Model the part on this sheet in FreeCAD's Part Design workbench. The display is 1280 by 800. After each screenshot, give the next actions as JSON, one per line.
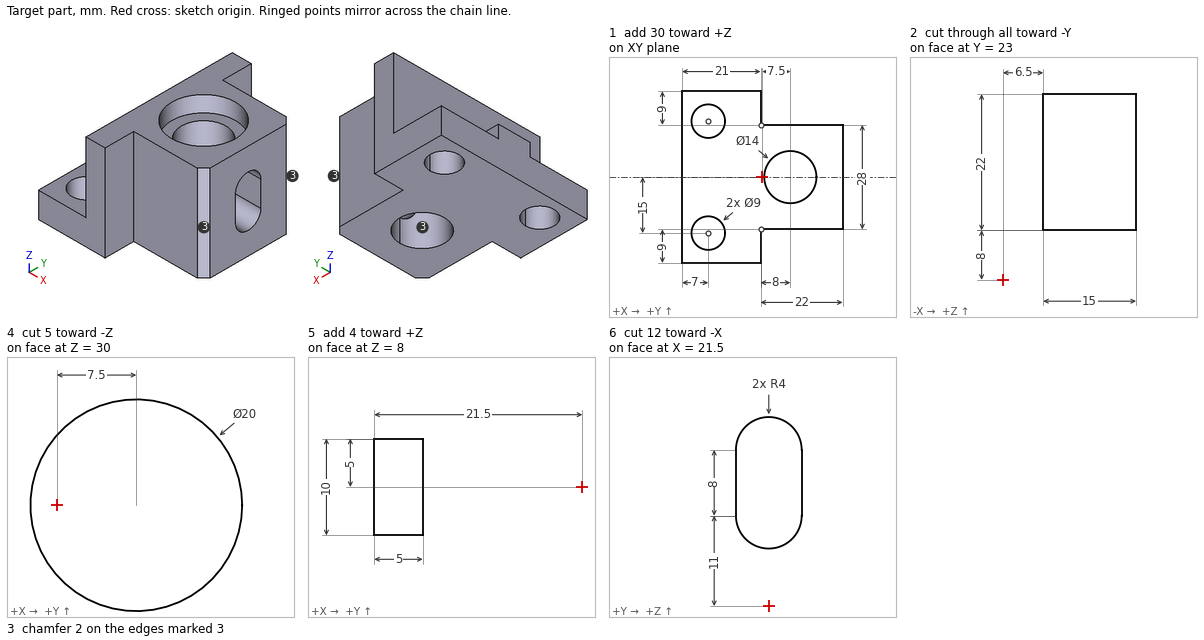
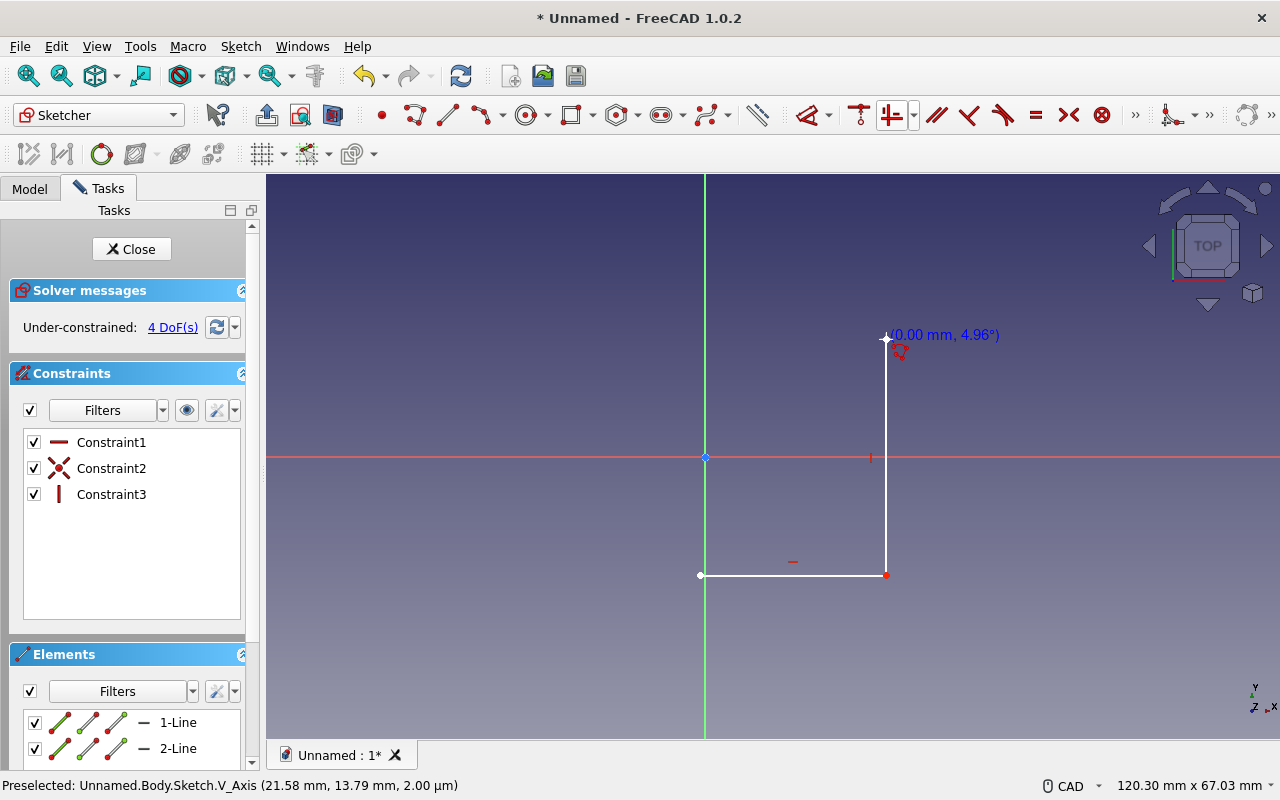
{"action": "scroll", "coordinate": [701, 339], "scroll_direction": "up", "scroll_amount": 7}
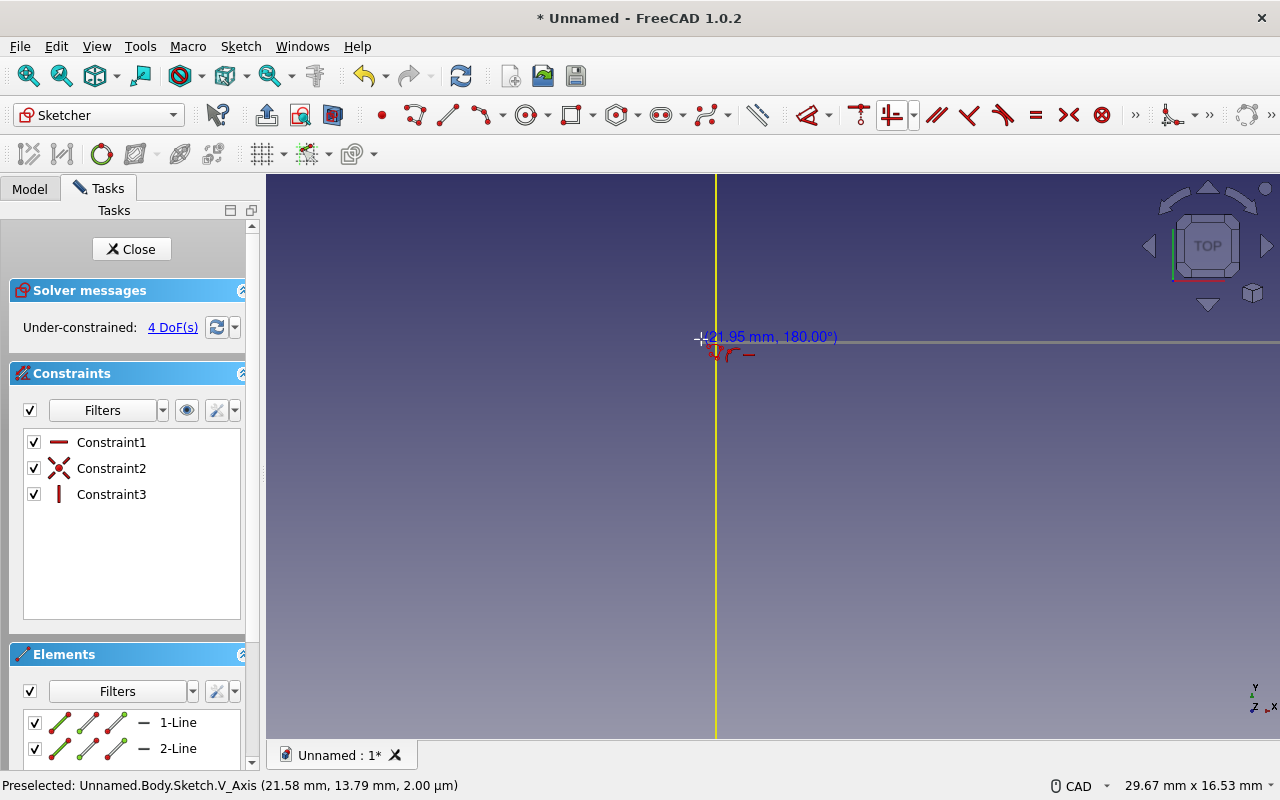
{"action": "left_click", "coordinate": [699, 338]}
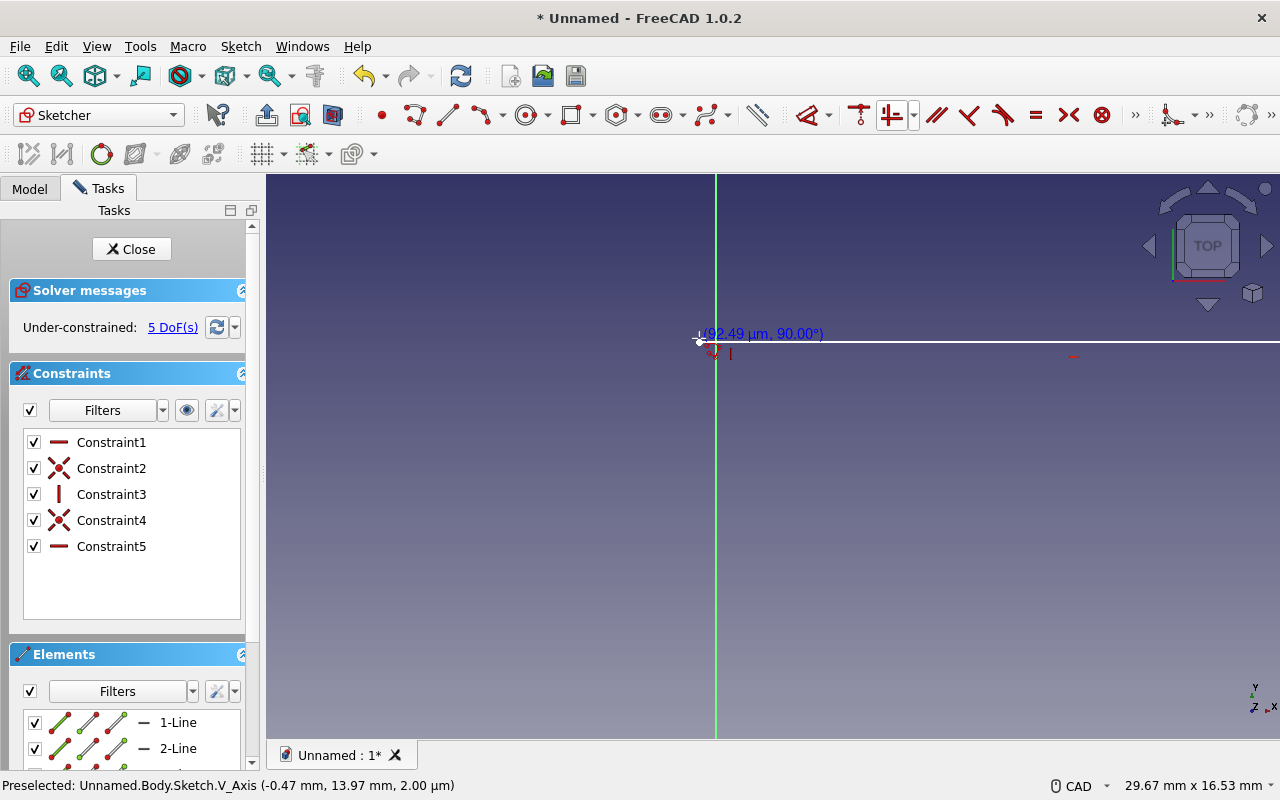
{"action": "scroll", "coordinate": [701, 338], "scroll_direction": "down", "scroll_amount": 7}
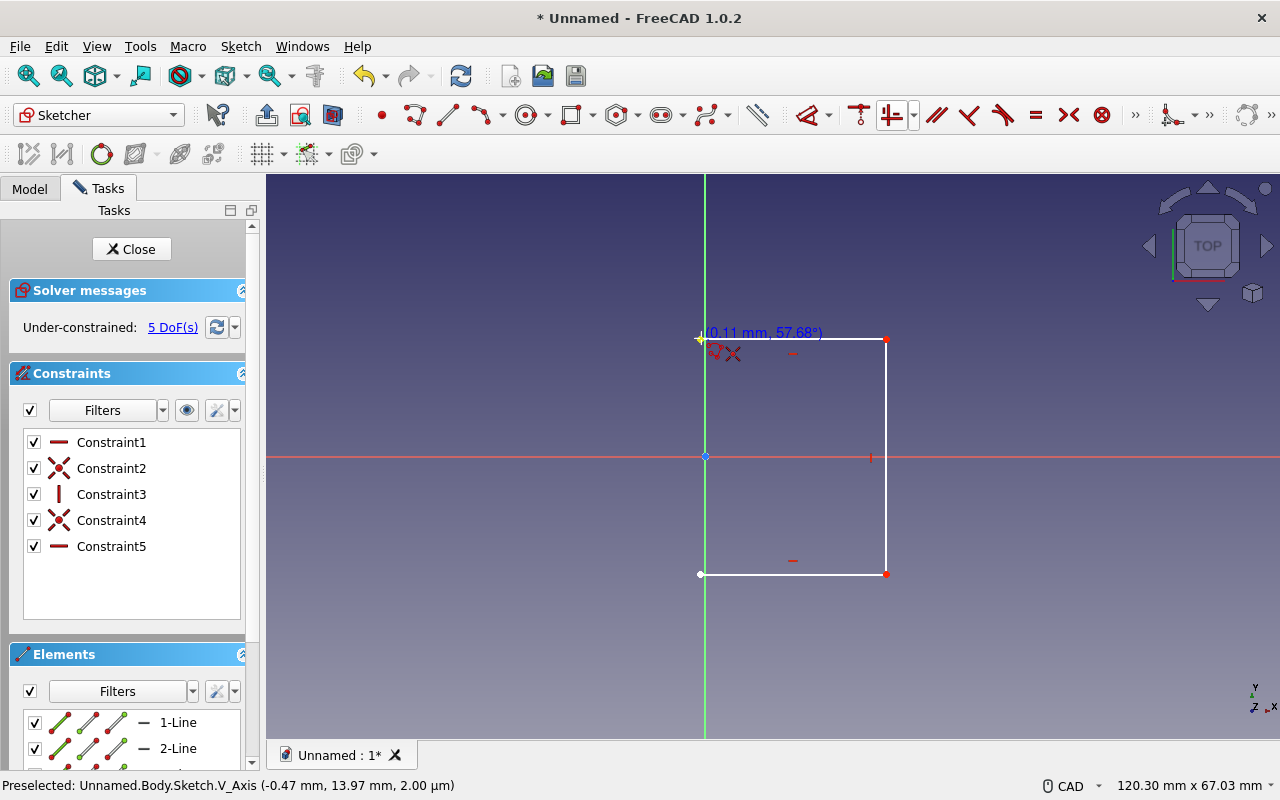
{"action": "scroll", "coordinate": [701, 263], "scroll_direction": "up", "scroll_amount": 7}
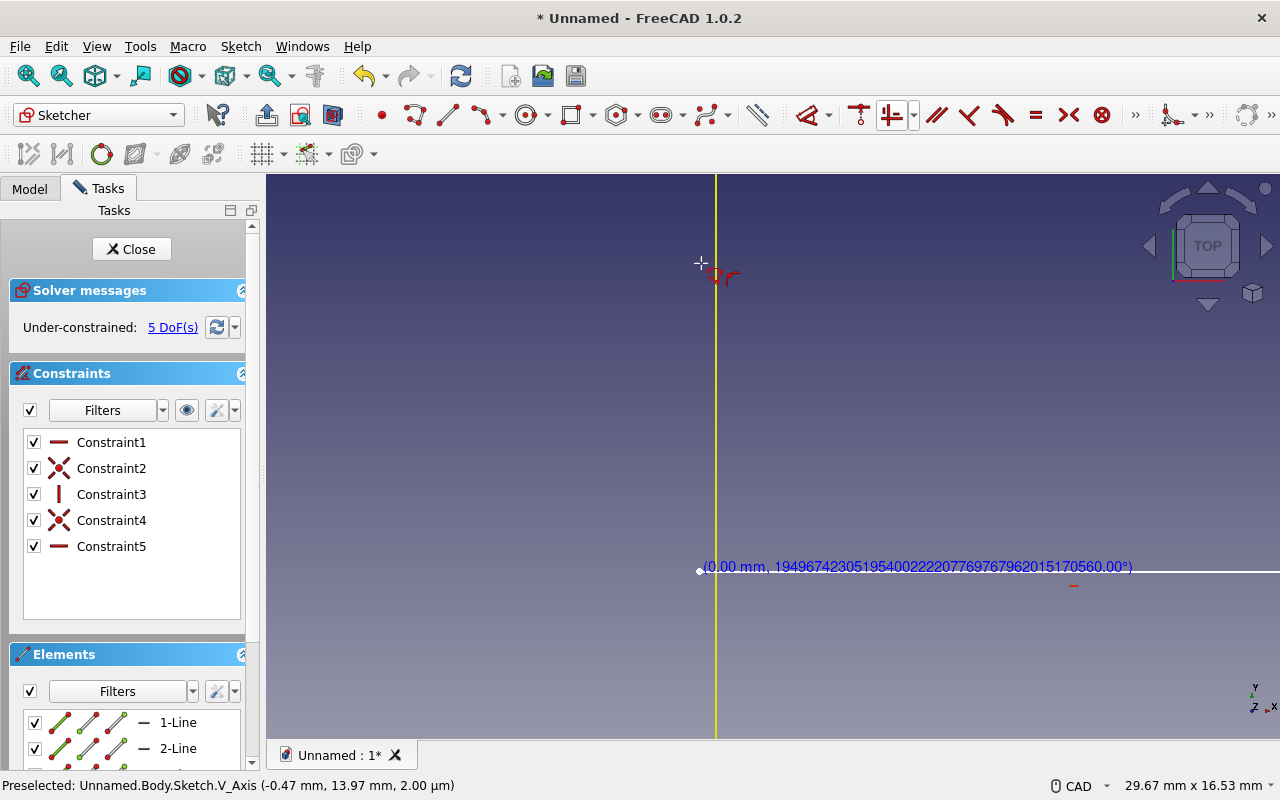
{"action": "left_click", "coordinate": [699, 261]}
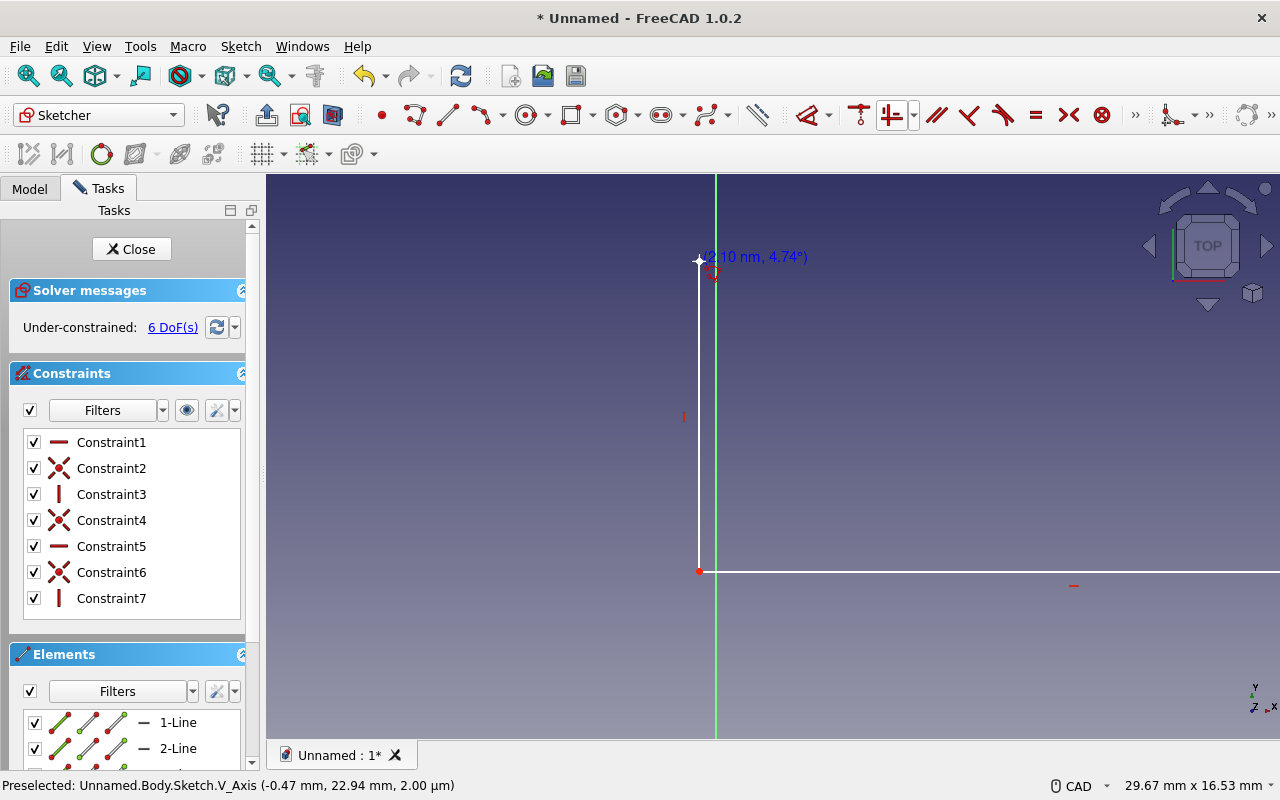
{"action": "scroll", "coordinate": [701, 263], "scroll_direction": "down", "scroll_amount": 7}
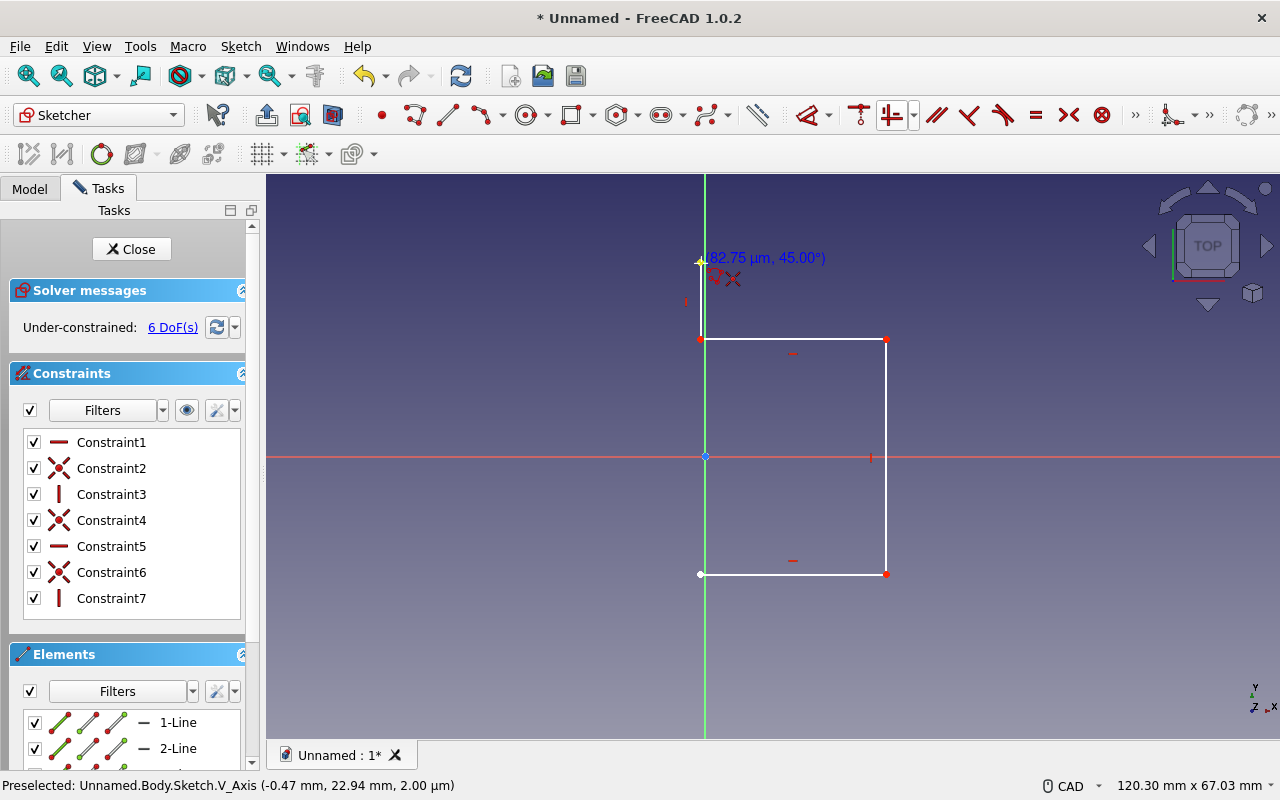
{"action": "left_click", "coordinate": [524, 263]}
{"action": "left_click", "coordinate": [524, 650]}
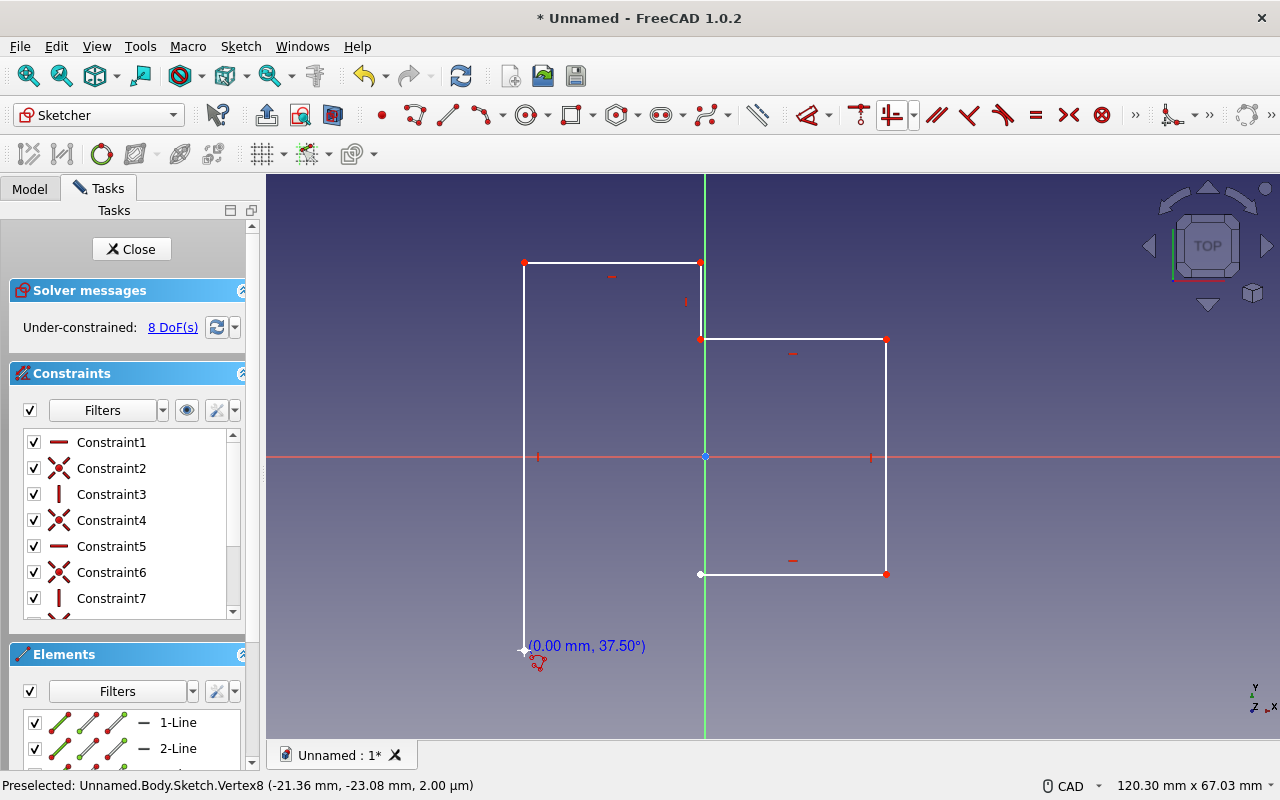
{"action": "scroll", "coordinate": [701, 650], "scroll_direction": "up", "scroll_amount": 7}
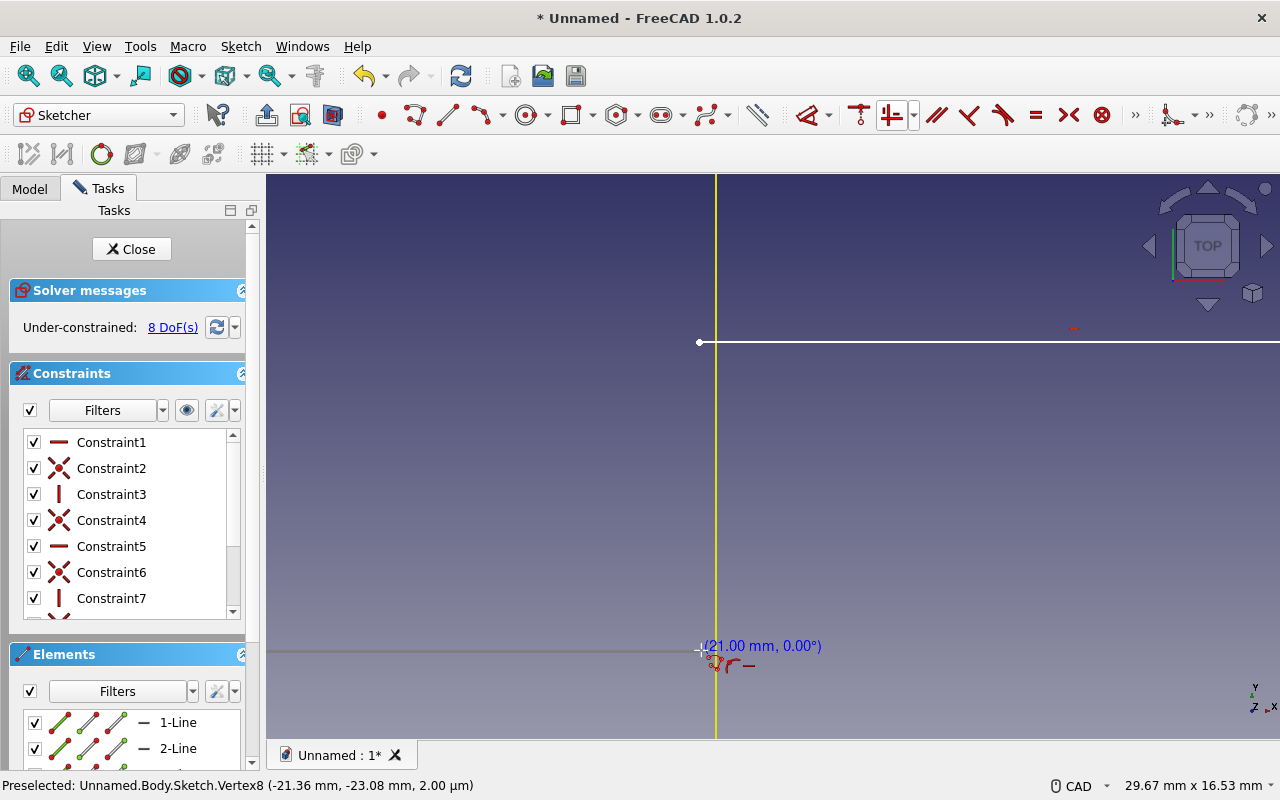
{"action": "left_click", "coordinate": [699, 647]}
{"action": "left_click", "coordinate": [699, 342]}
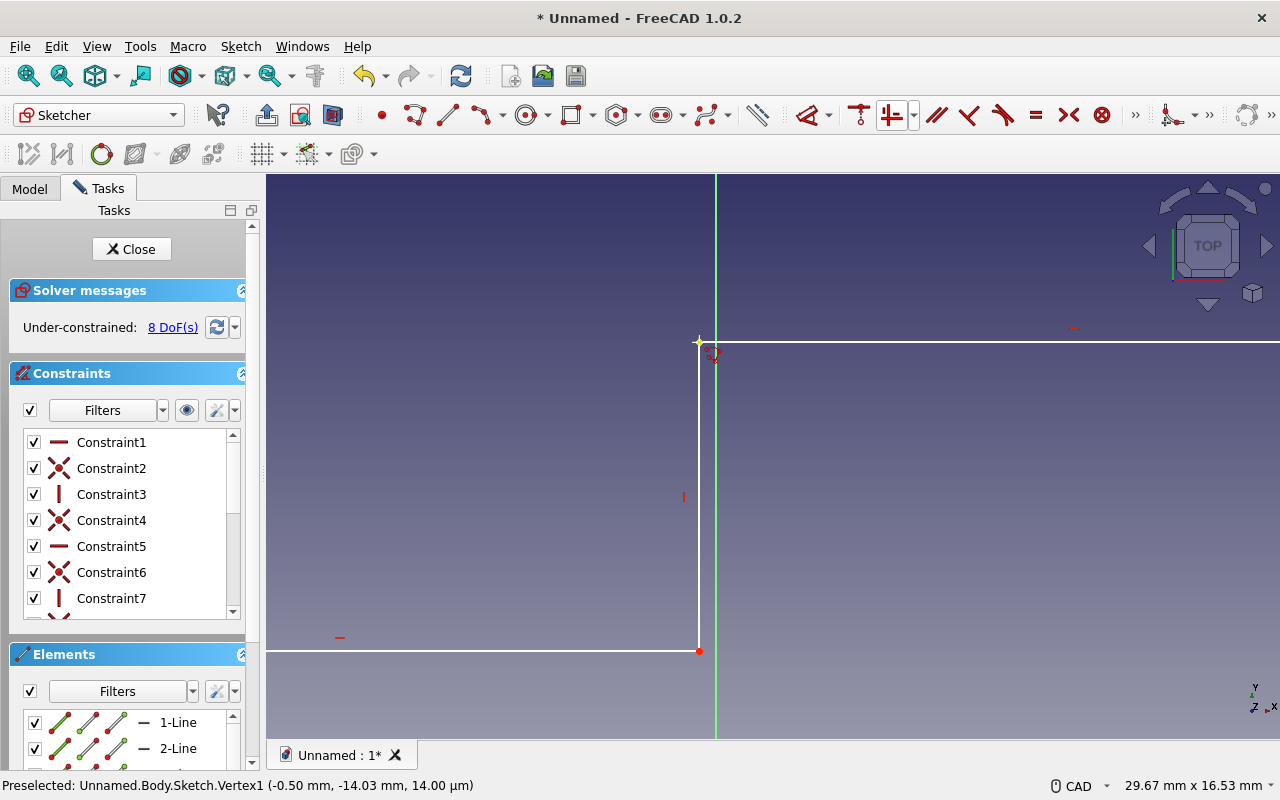
{"action": "key", "text": "g c"}